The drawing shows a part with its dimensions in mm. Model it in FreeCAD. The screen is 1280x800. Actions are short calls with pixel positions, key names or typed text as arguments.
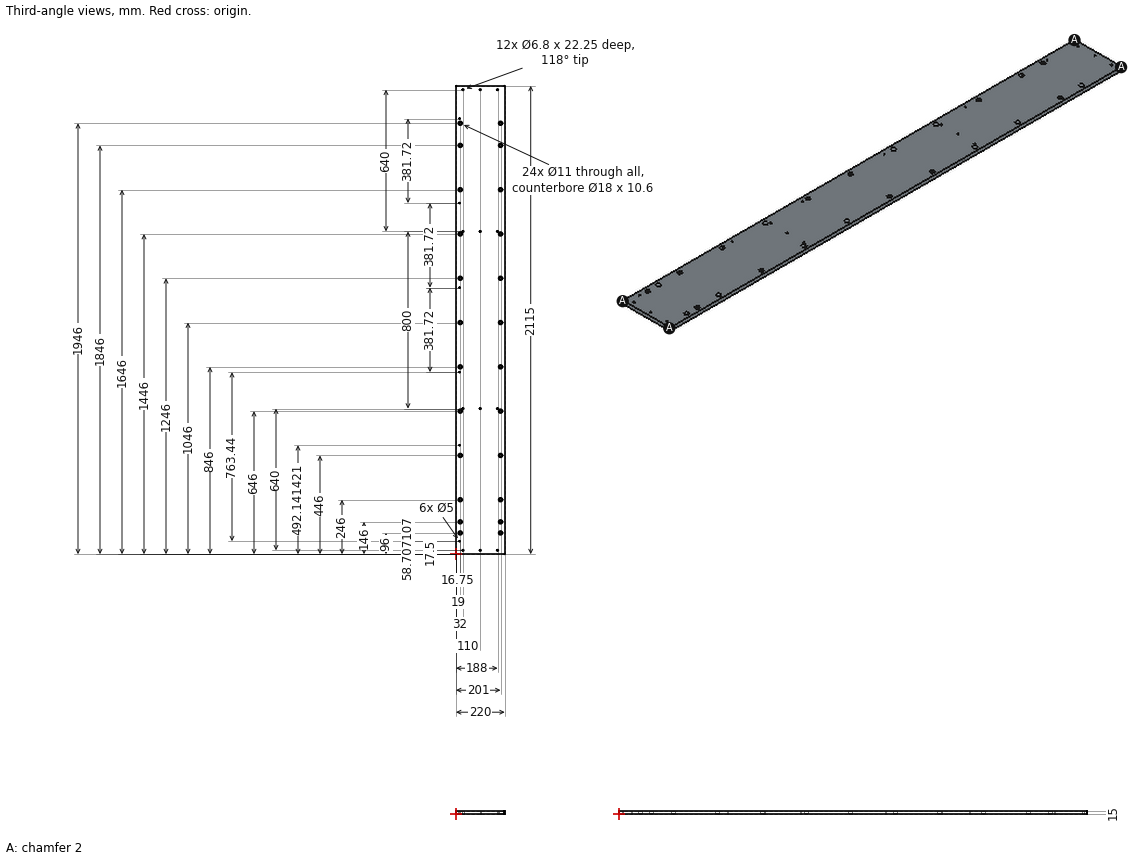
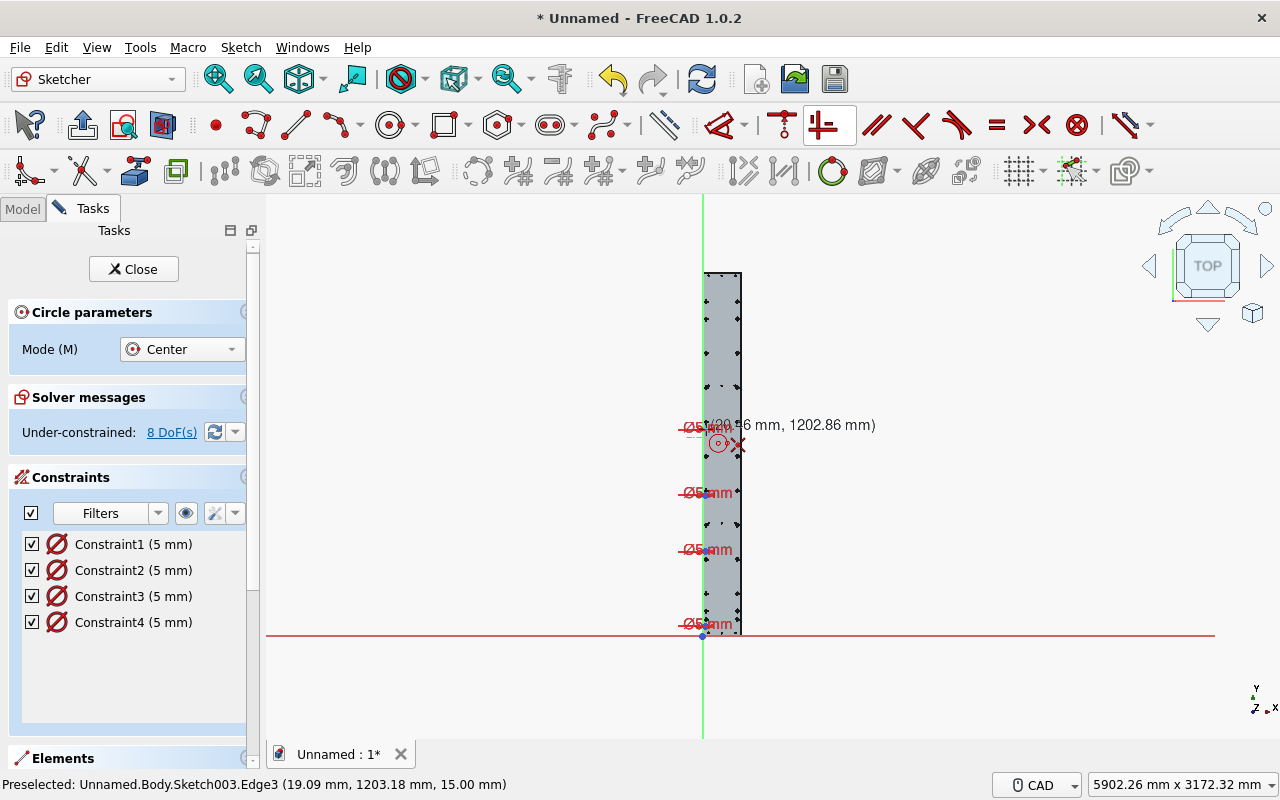
scroll(706, 364, up, 20)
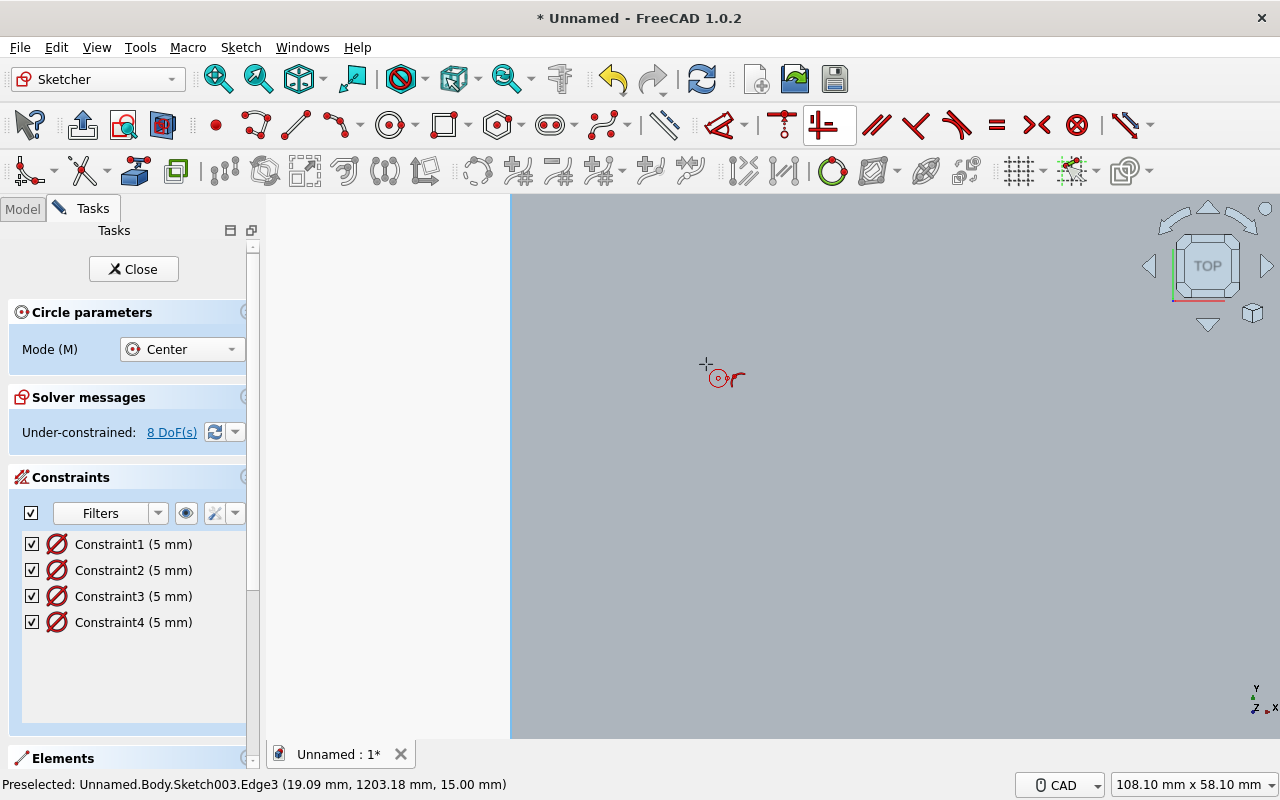
scroll(704, 466, down, 15)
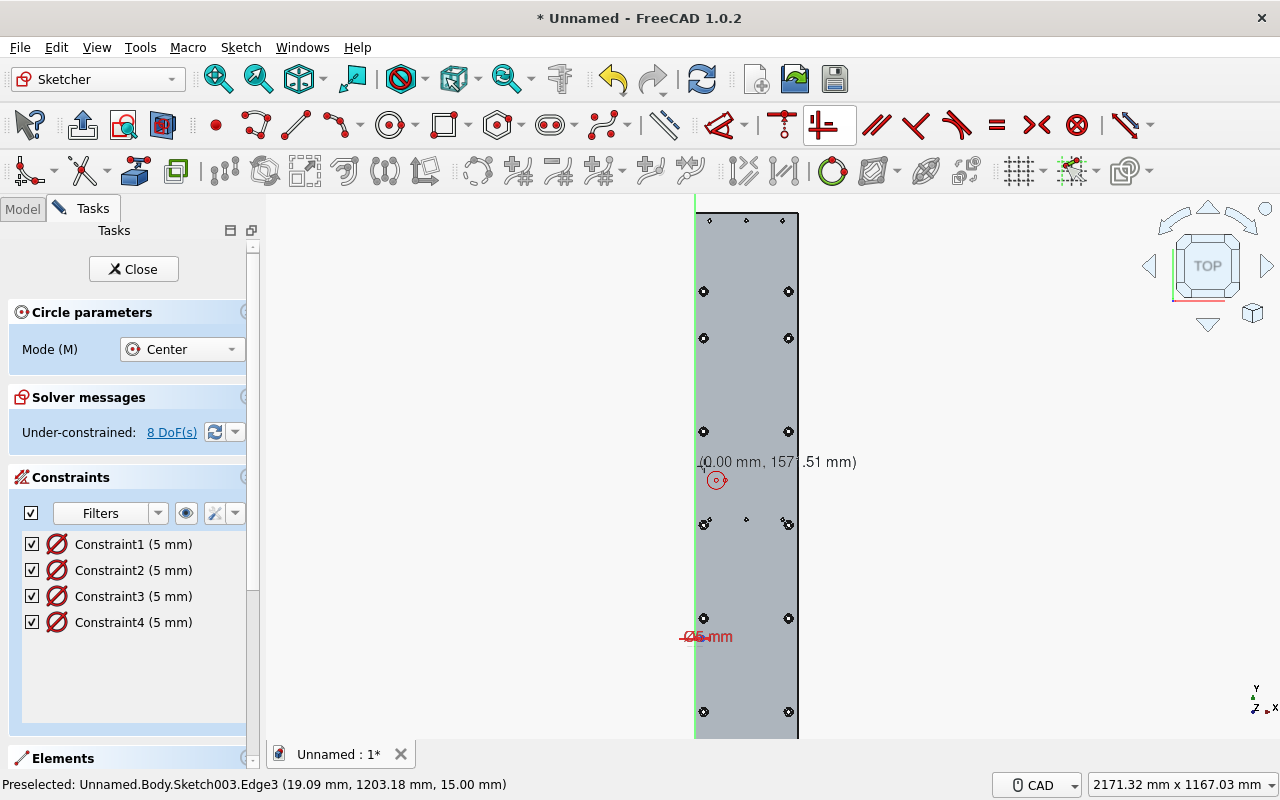
scroll(708, 307, down, 5)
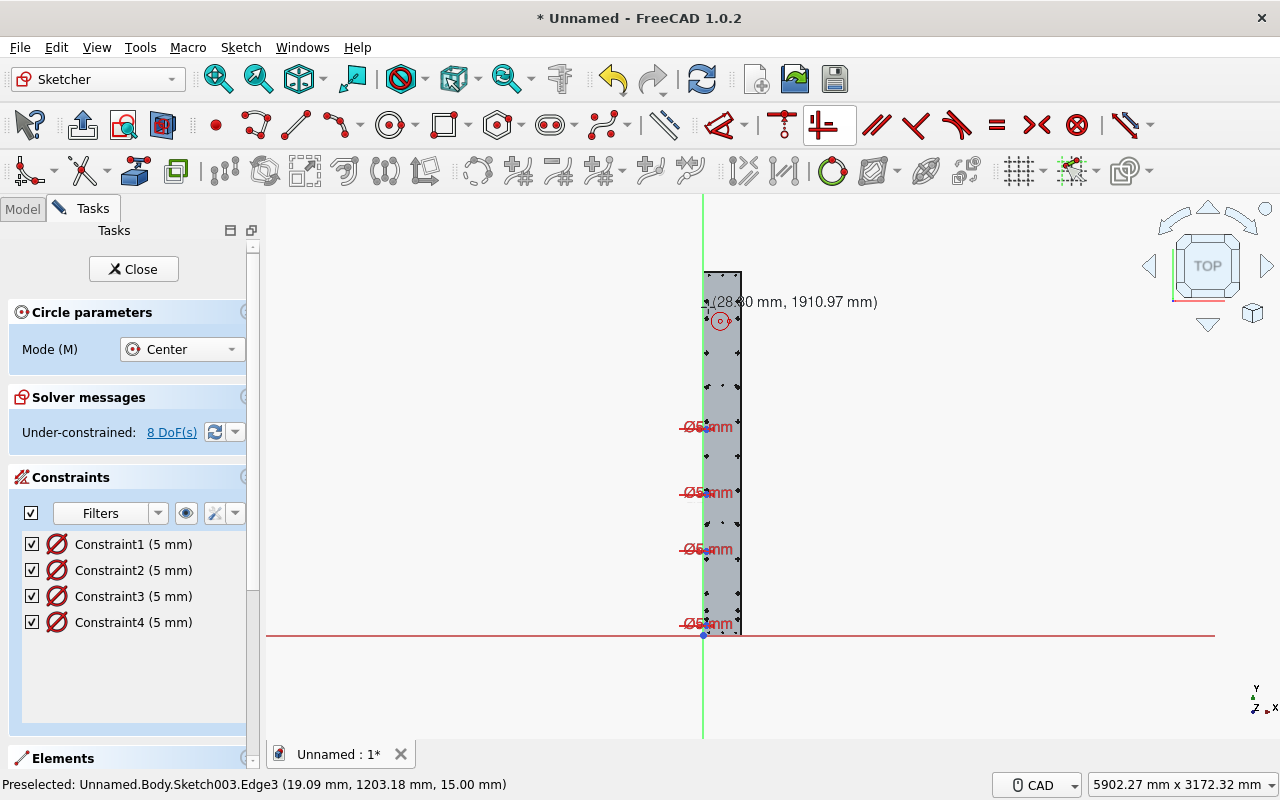
scroll(706, 363, up, 9)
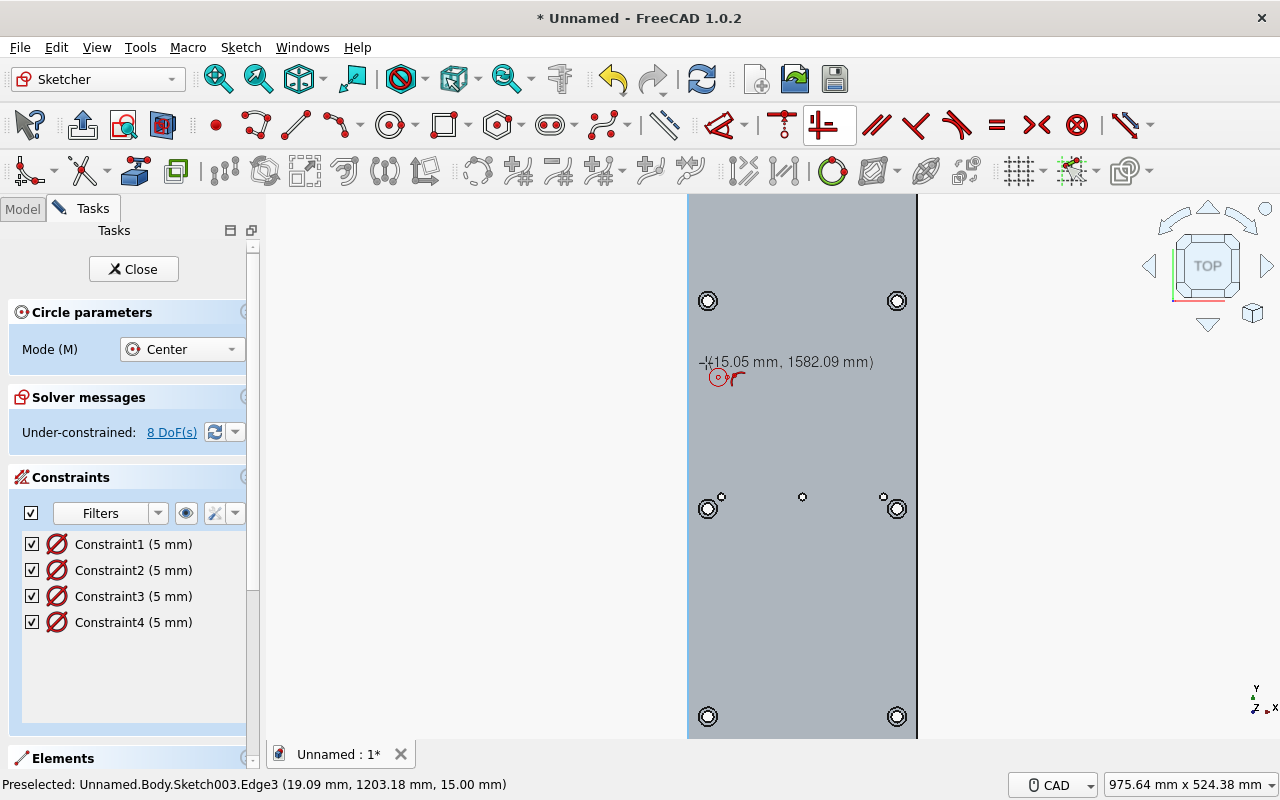
click(706, 364)
move(707, 362)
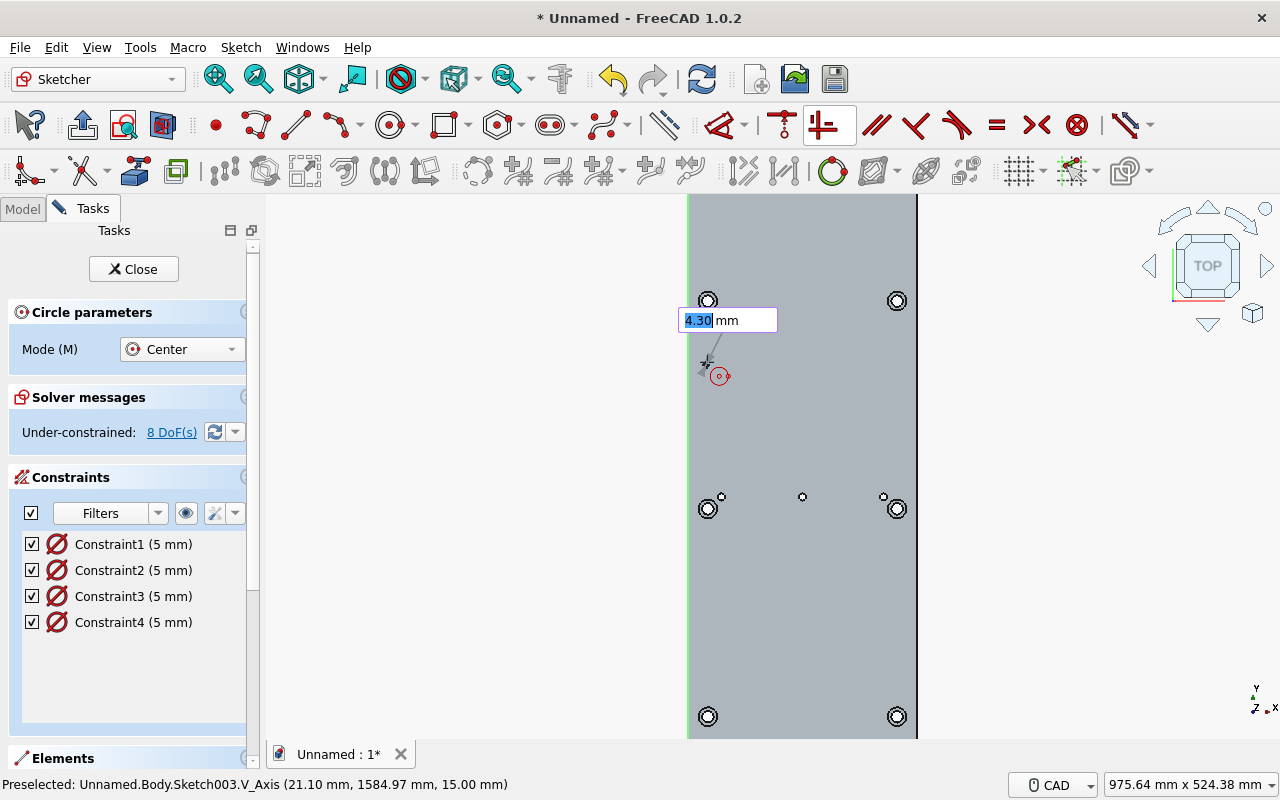
text(5)
key(Return)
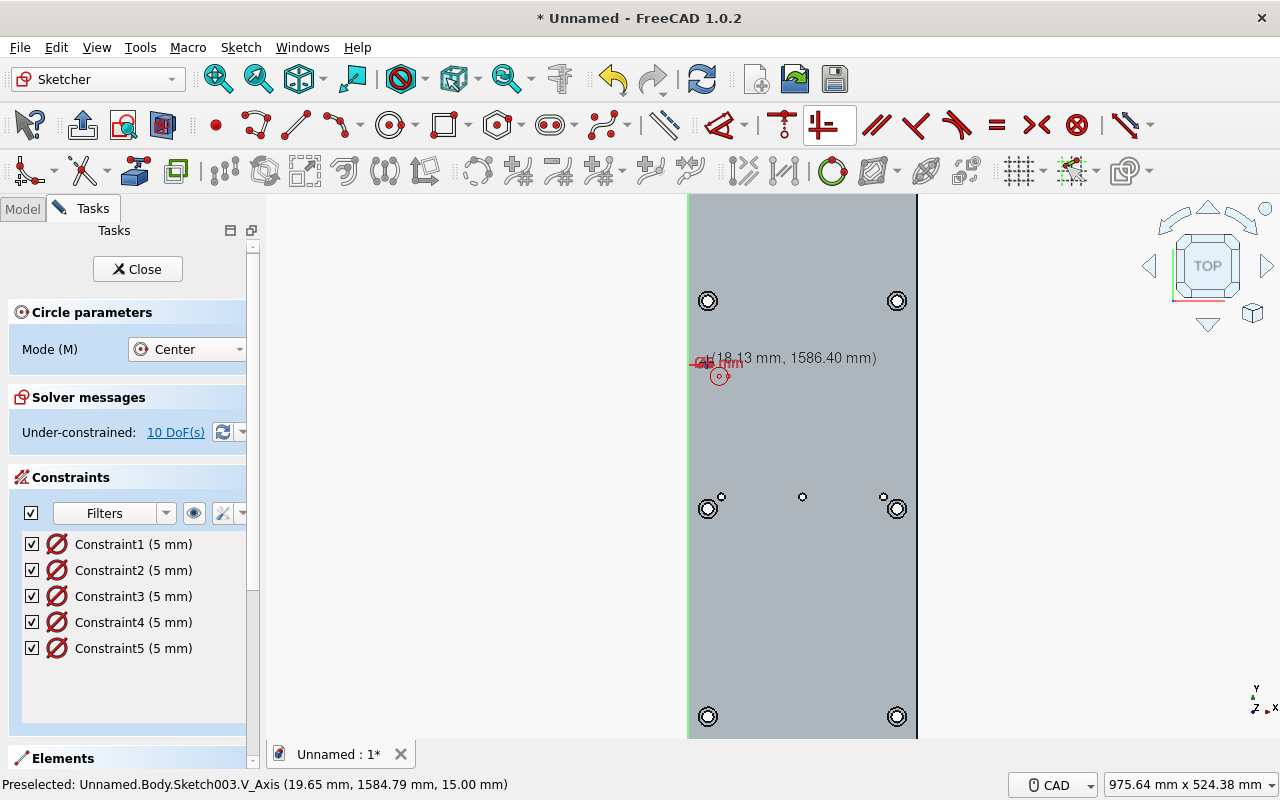
scroll(706, 363, down, 9)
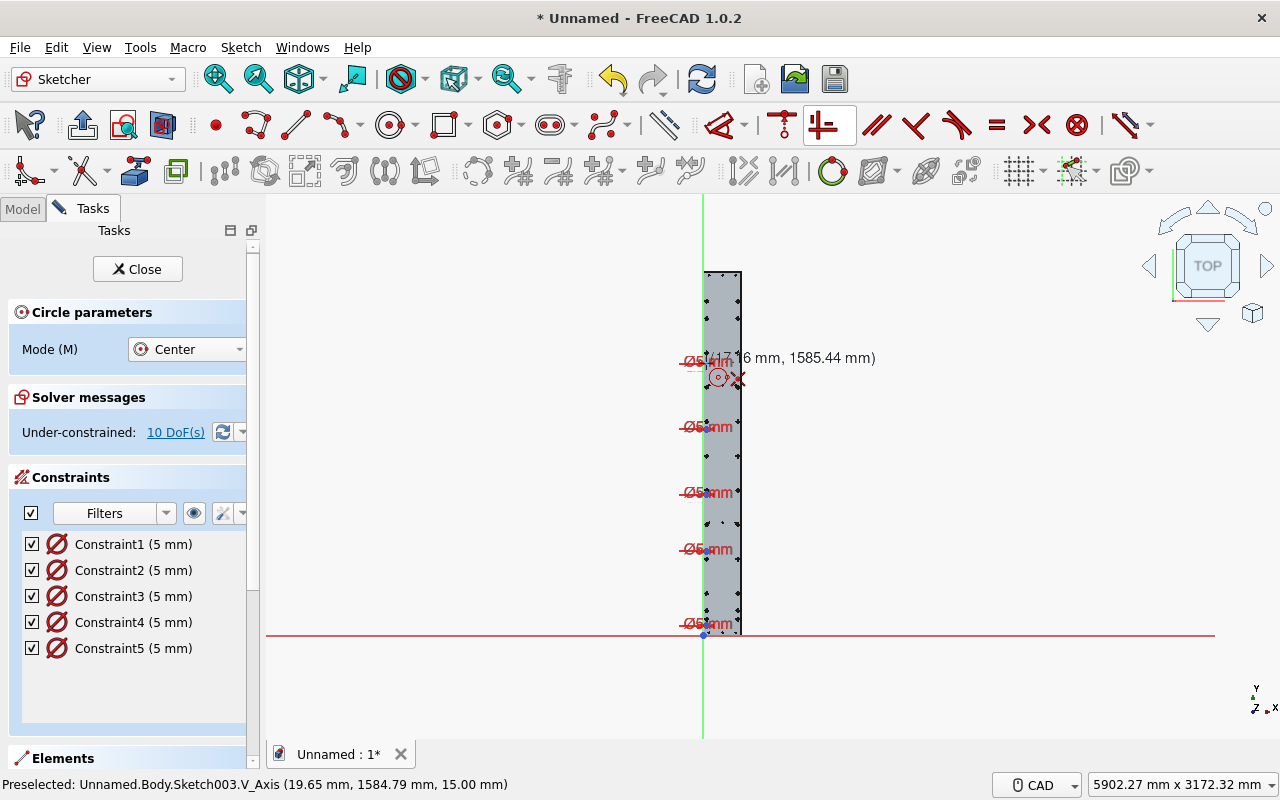
scroll(706, 298, up, 20)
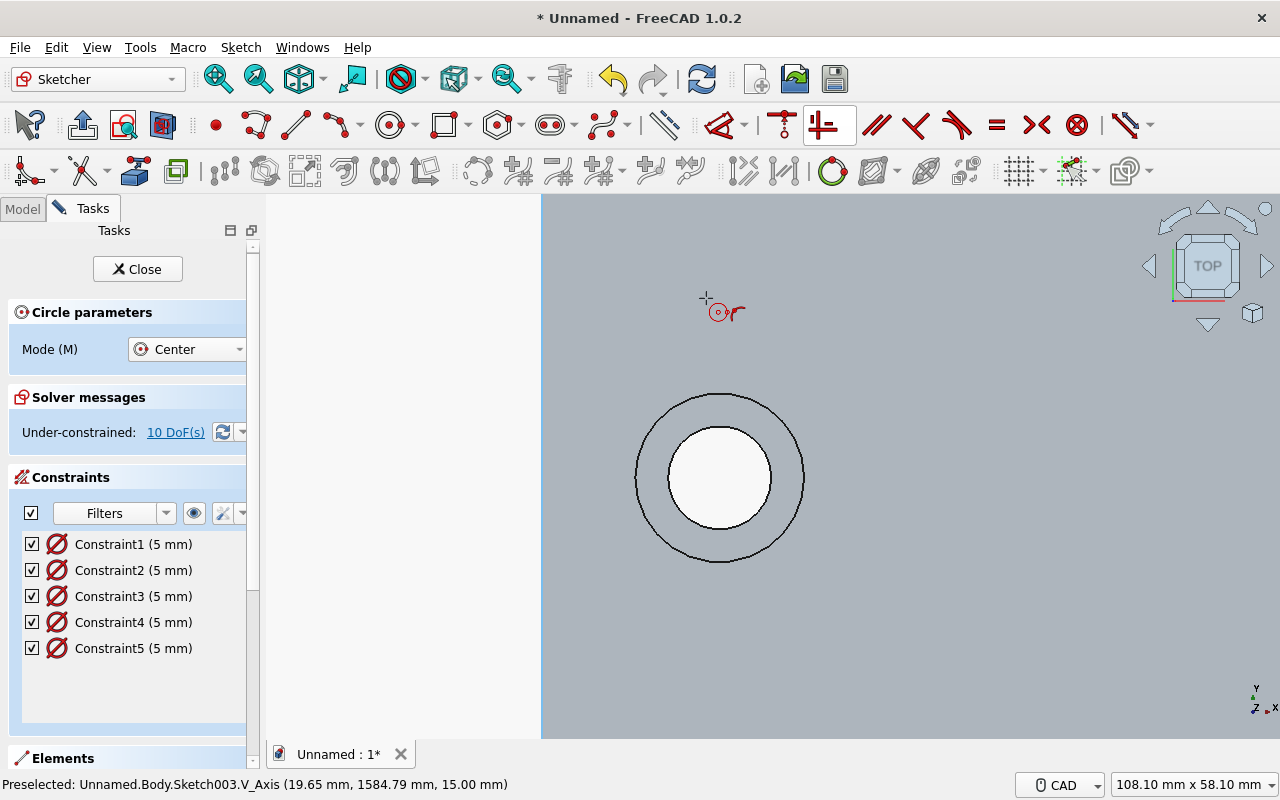
scroll(704, 466, down, 15)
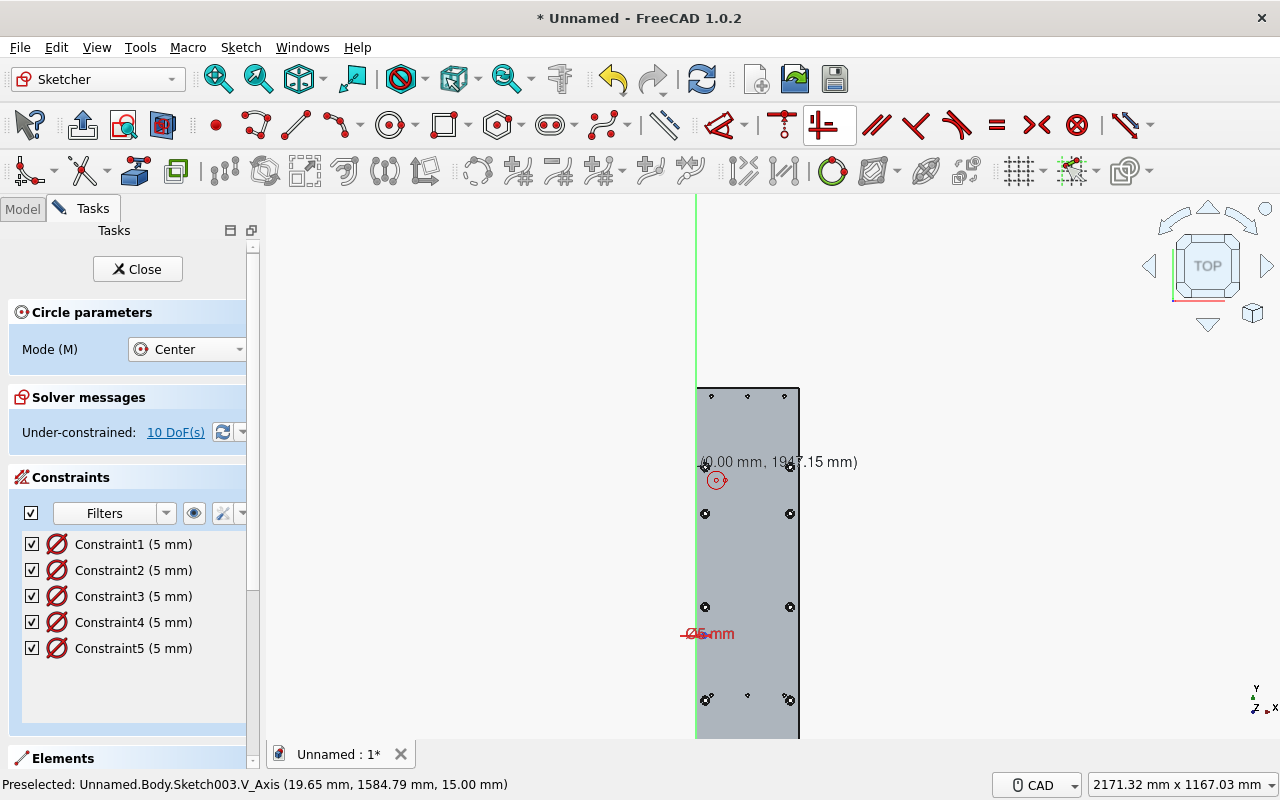
scroll(707, 222, down, 5)